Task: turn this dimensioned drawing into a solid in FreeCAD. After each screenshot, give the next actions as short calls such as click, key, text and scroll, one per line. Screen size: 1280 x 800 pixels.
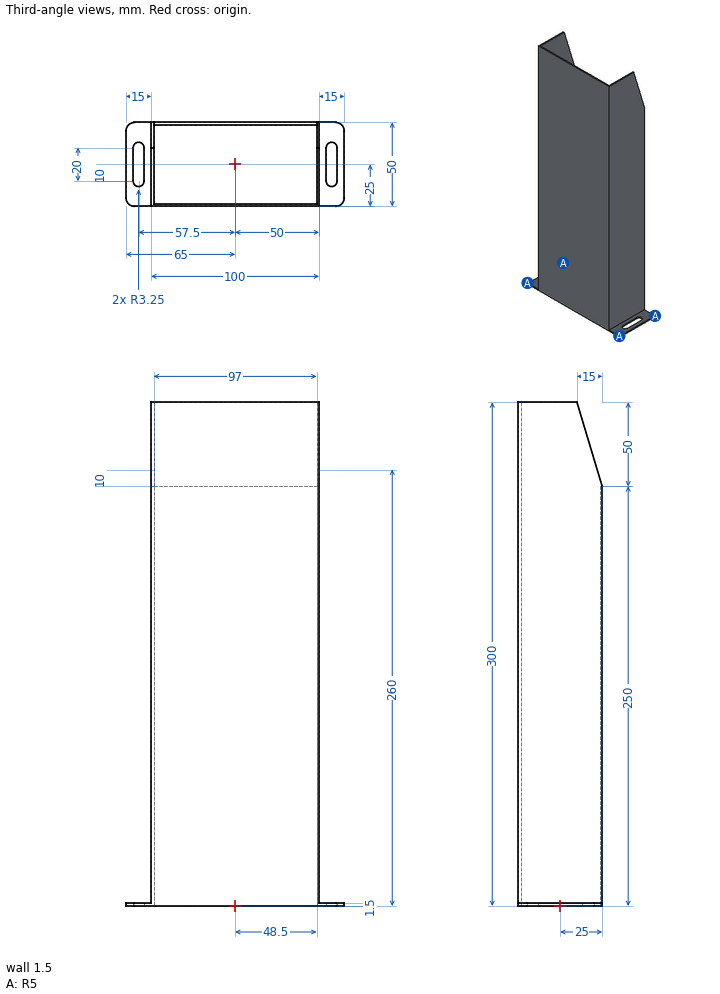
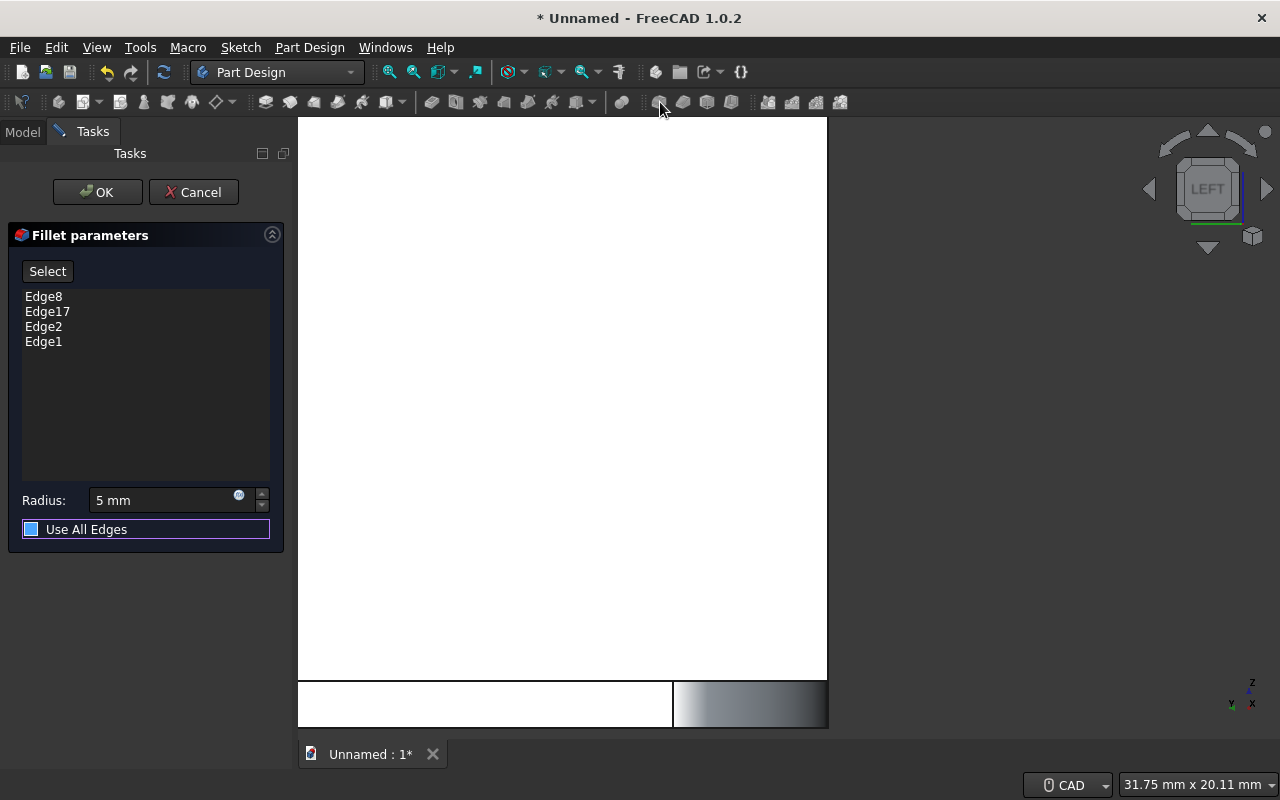
click(98, 192)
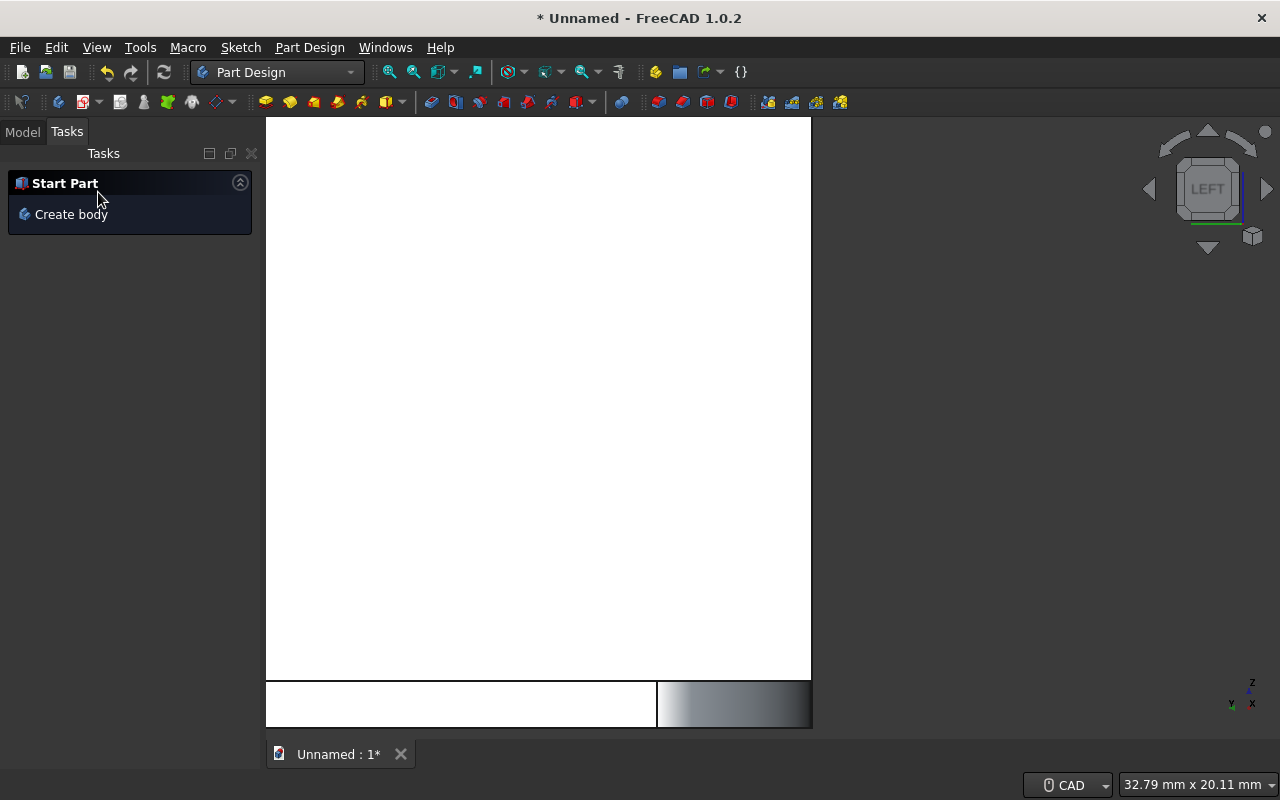
click(390, 72)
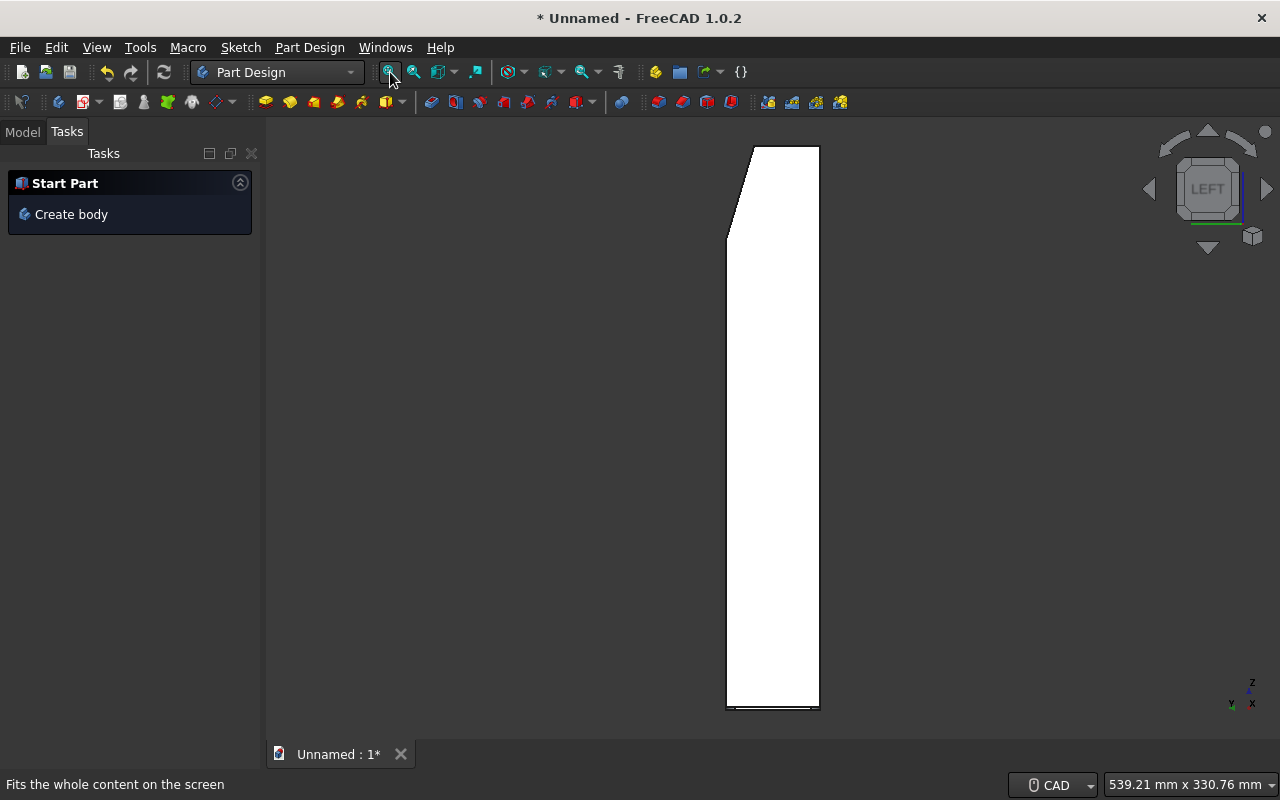
key(0)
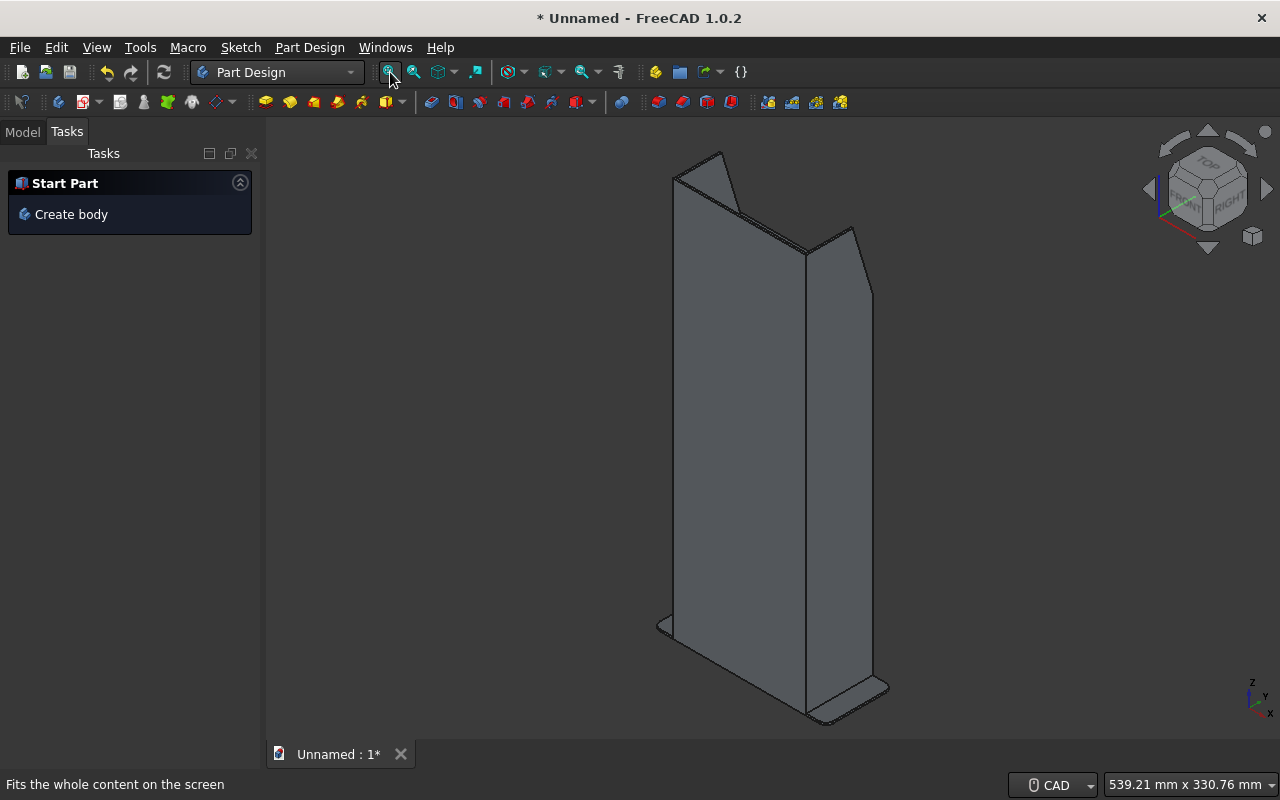
key(2)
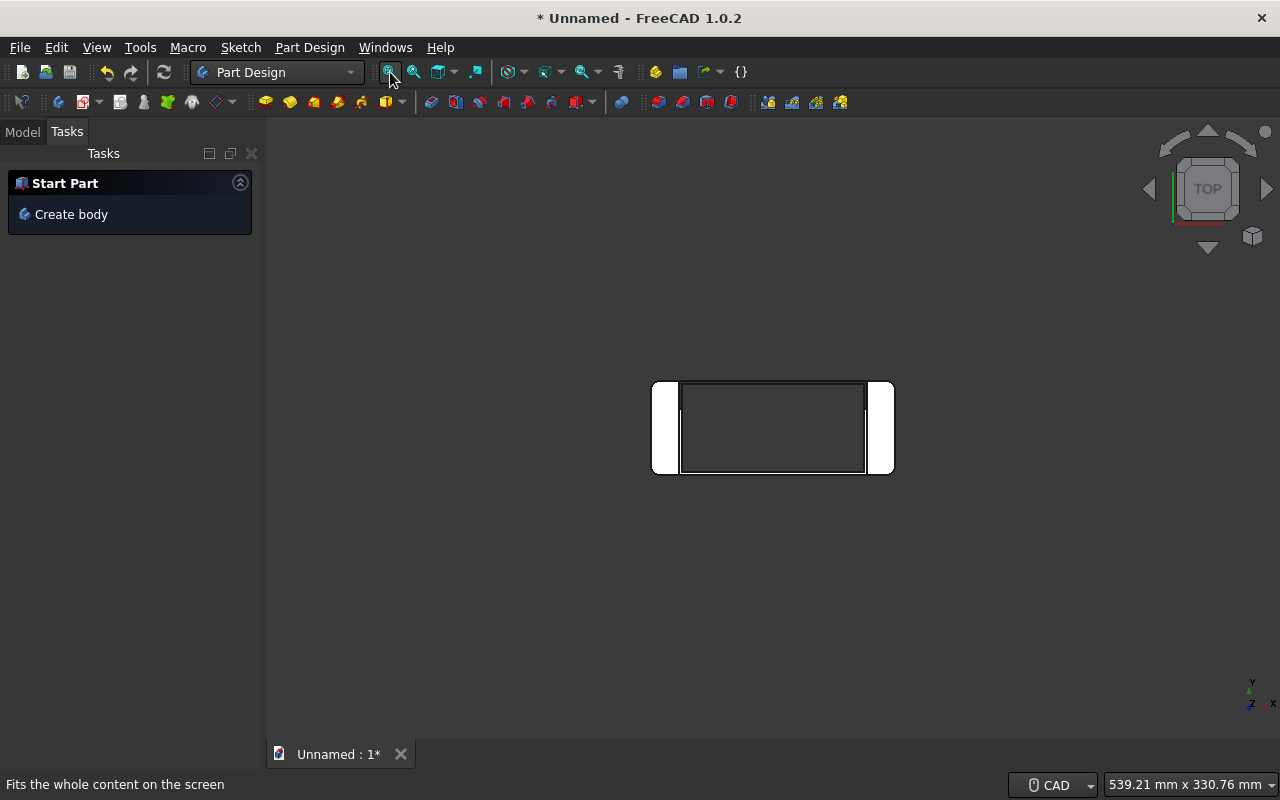
click(390, 72)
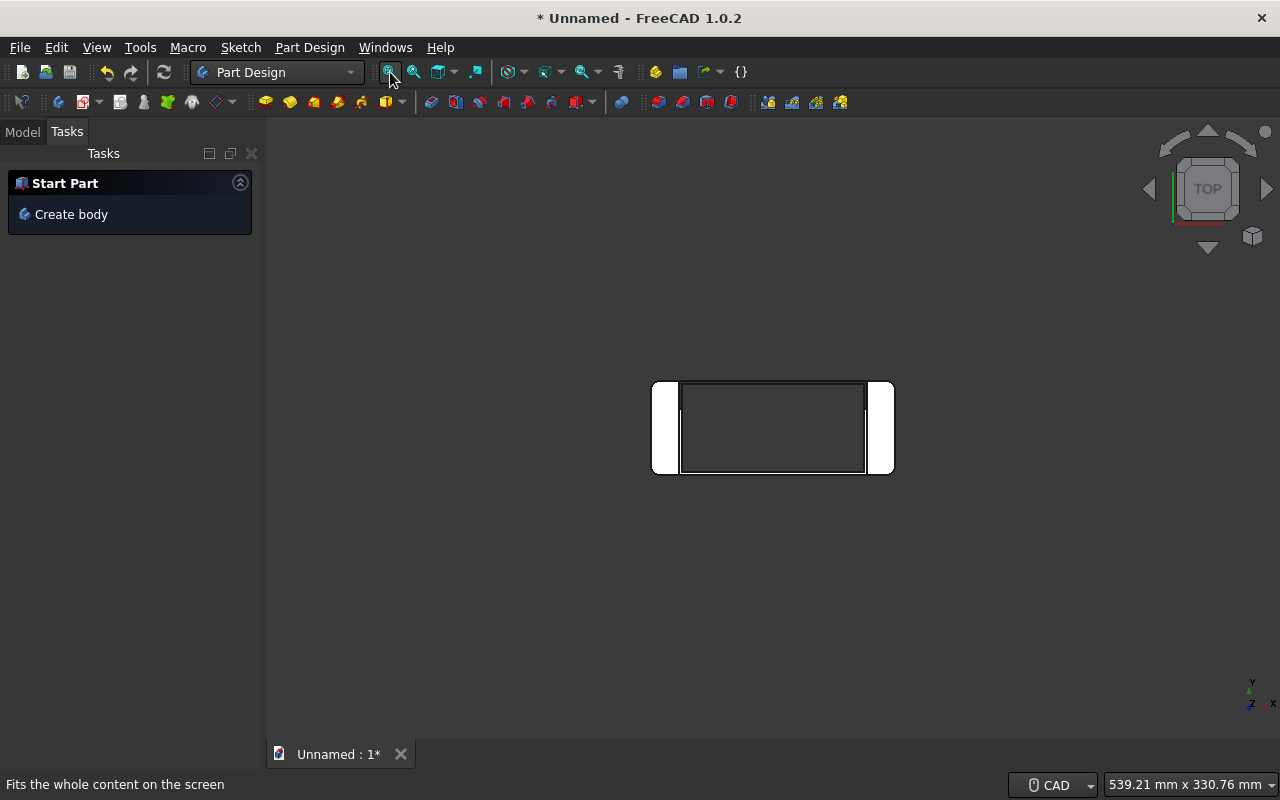
click(665, 400)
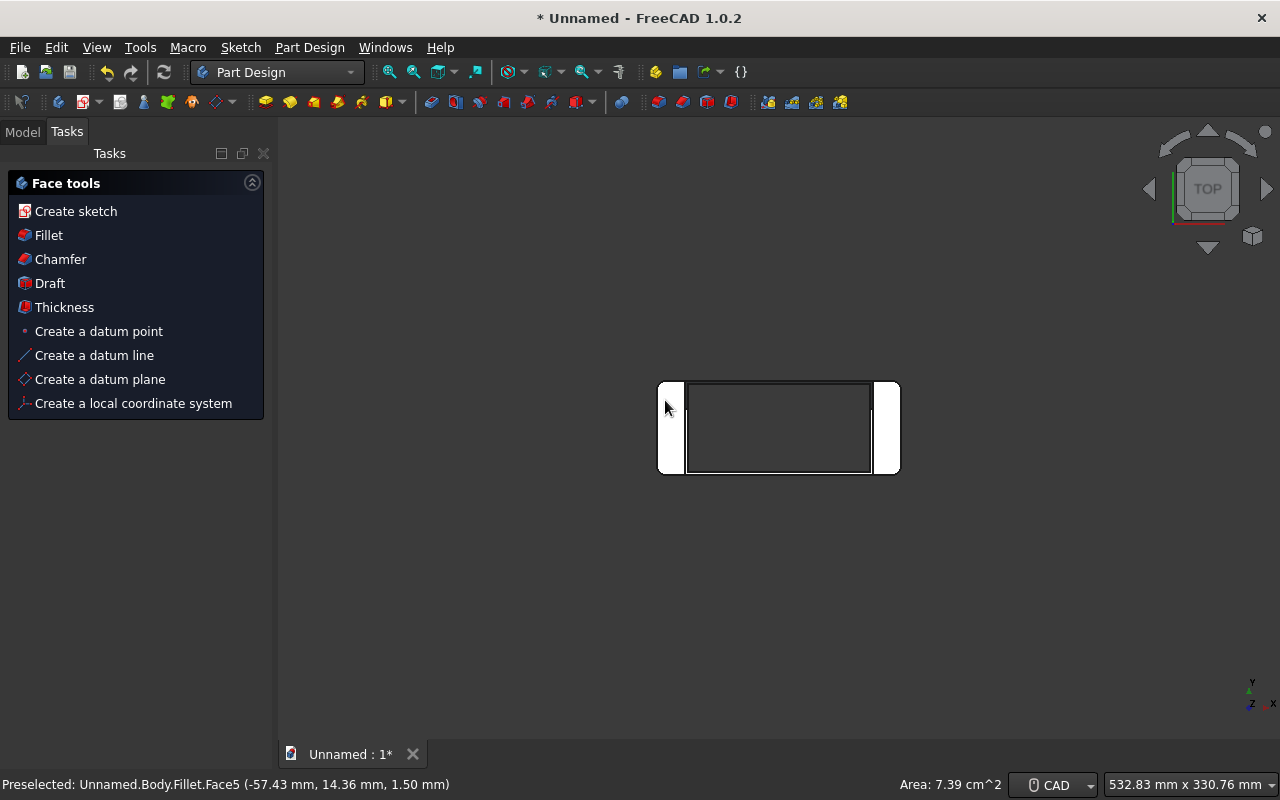
click(84, 102)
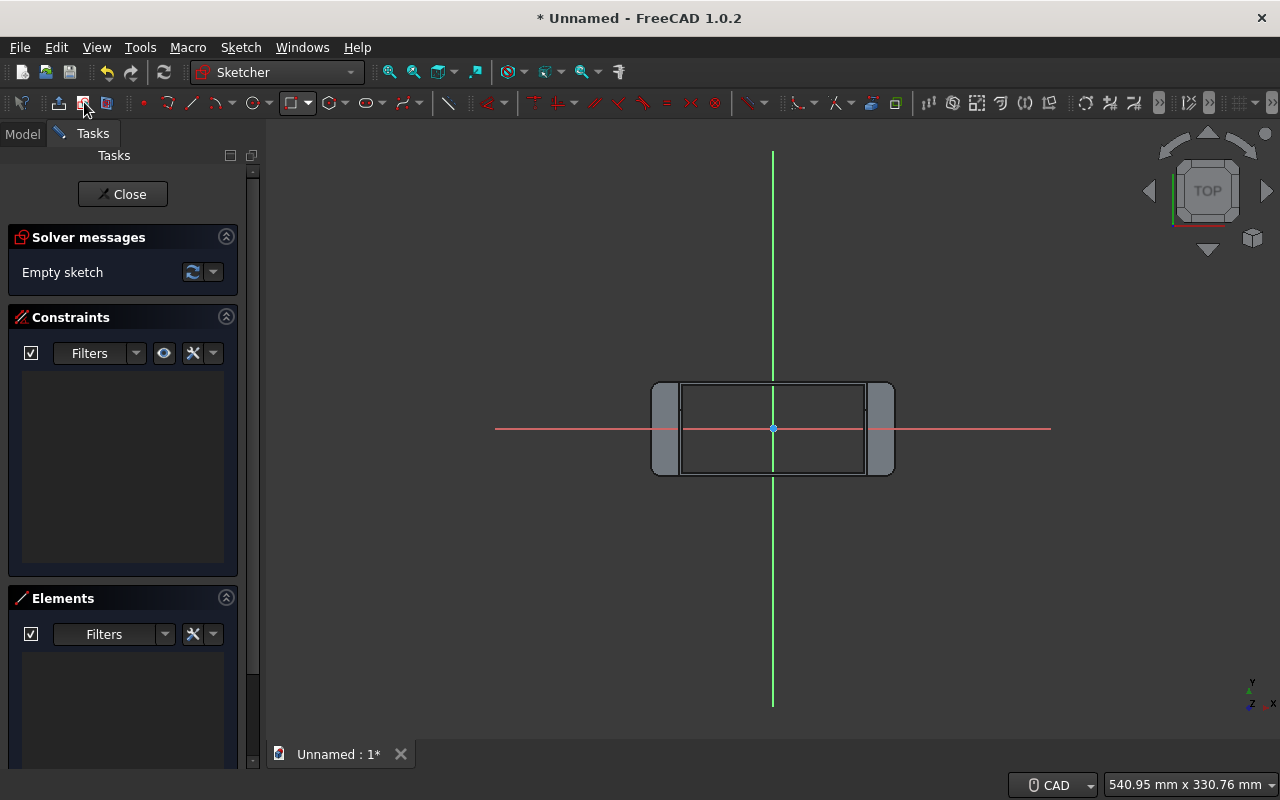
scroll(719, 429, up, 8)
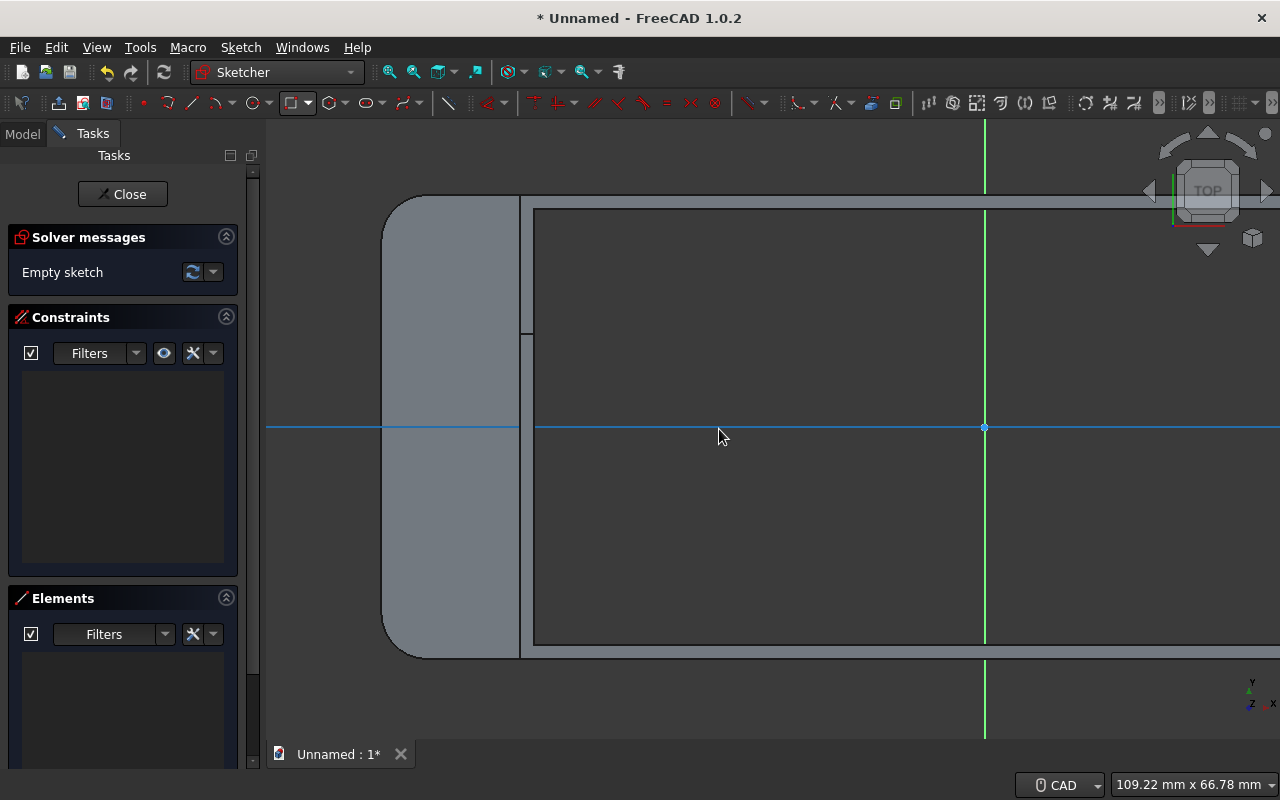
click(366, 104)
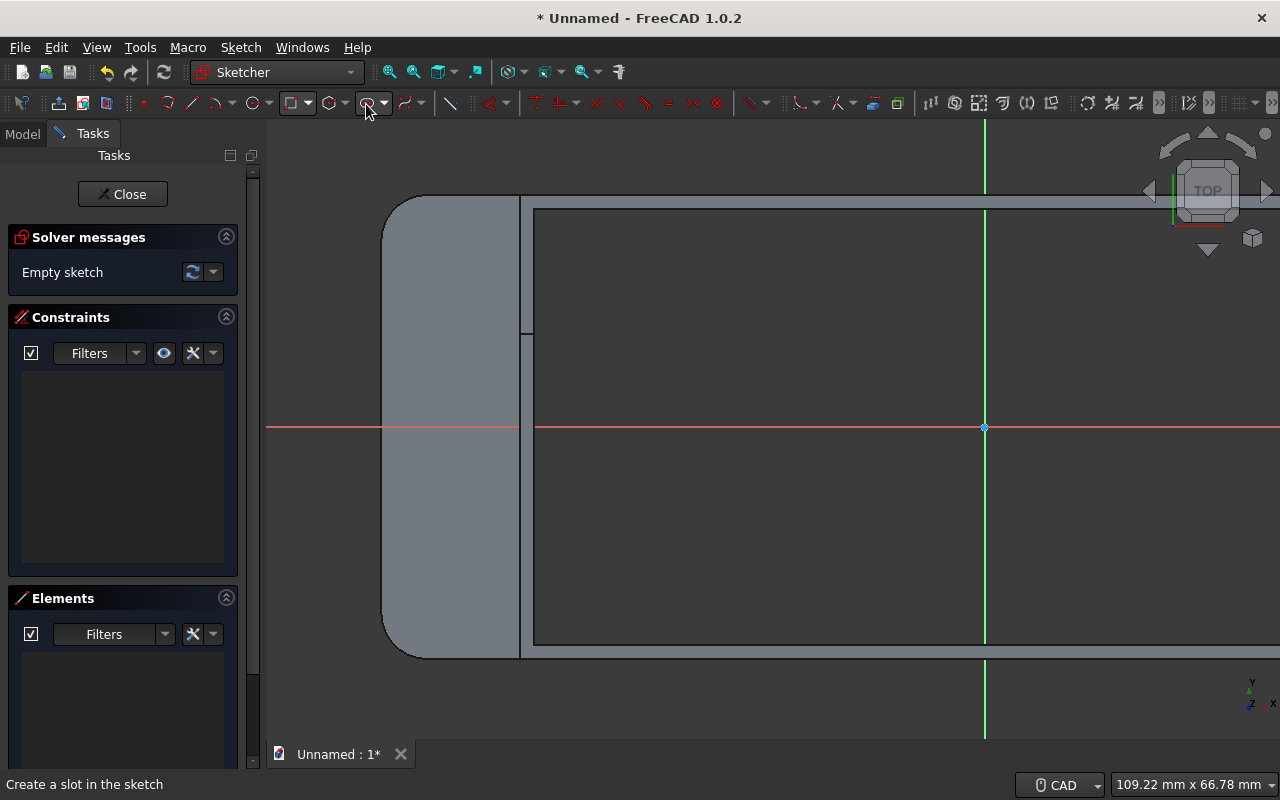
click(451, 520)